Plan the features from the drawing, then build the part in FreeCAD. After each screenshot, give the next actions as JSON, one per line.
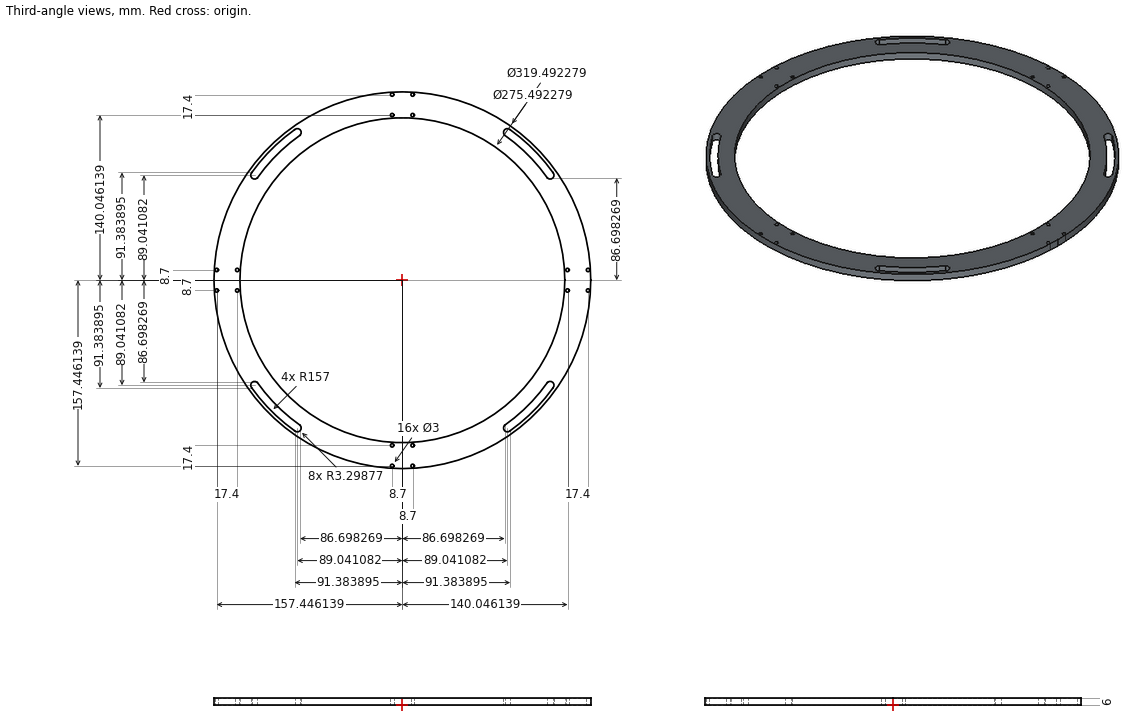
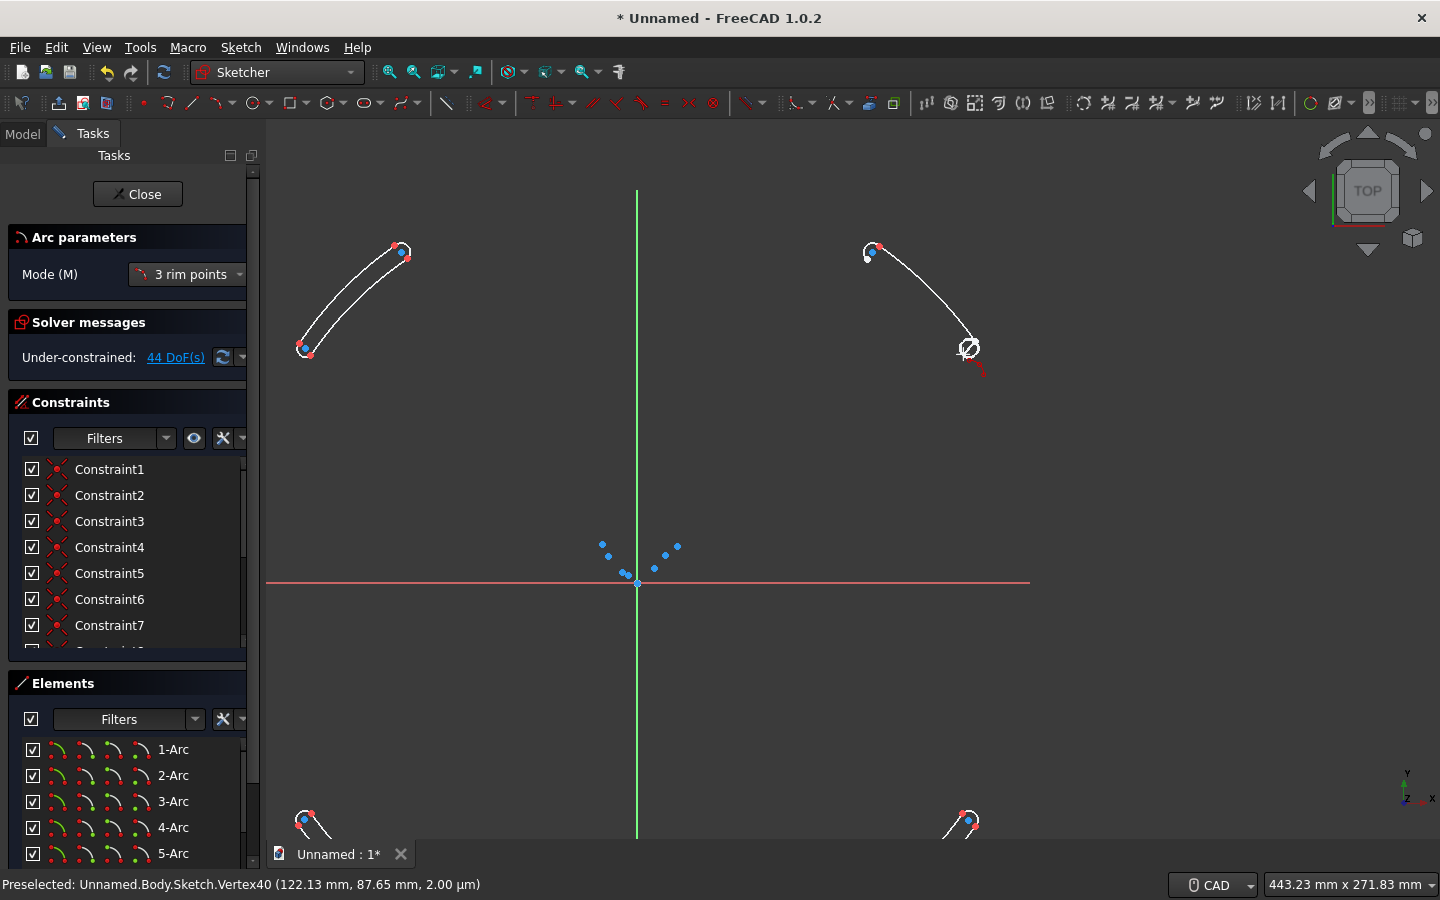
{"action": "scroll", "coordinate": [975, 354], "scroll_direction": "up", "scroll_amount": 3}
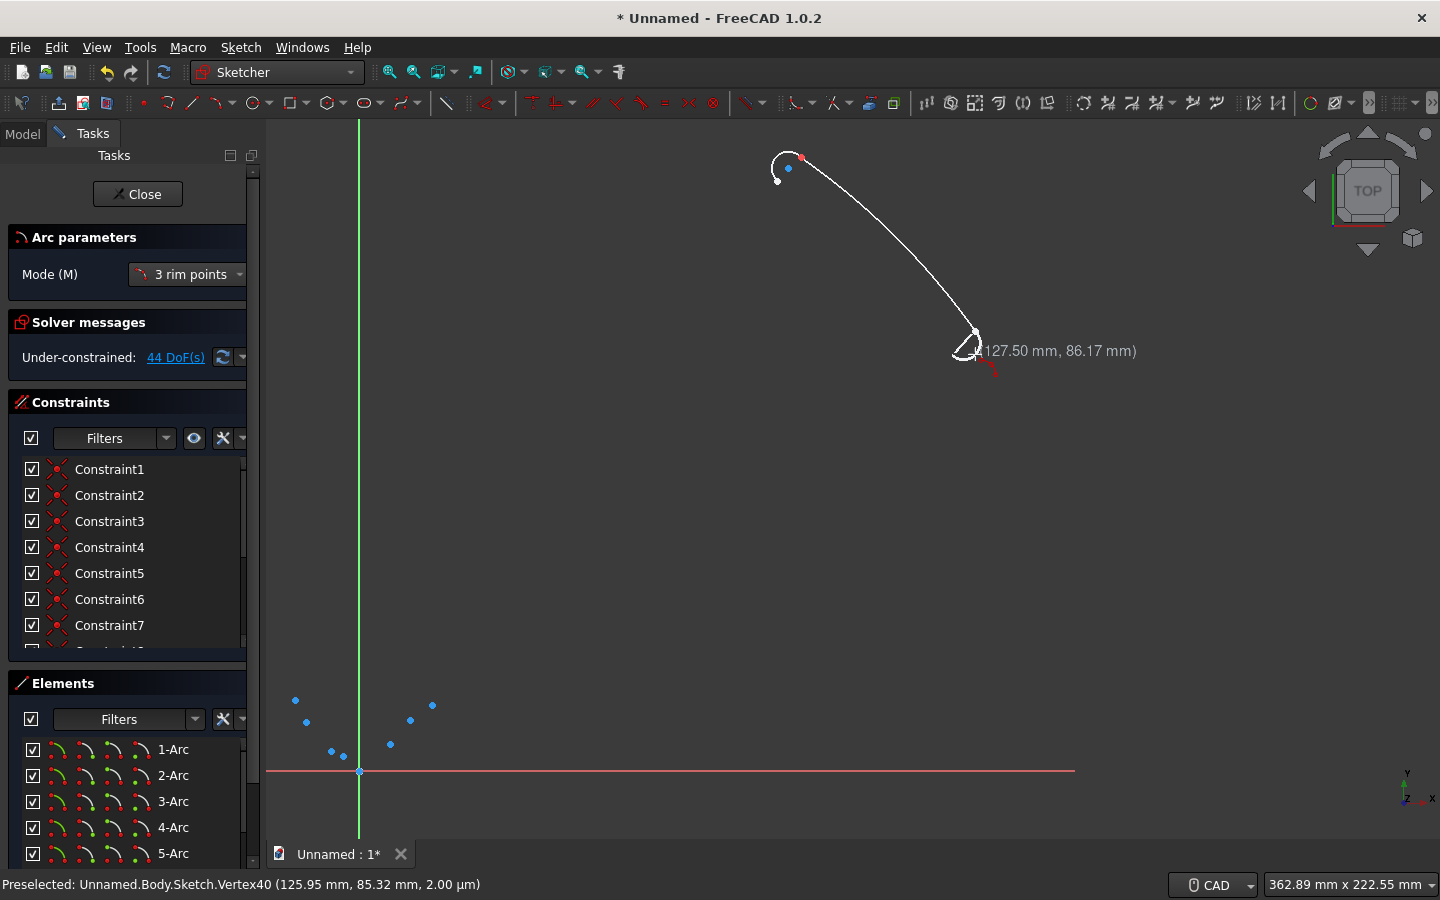
{"action": "left_click", "coordinate": [975, 353]}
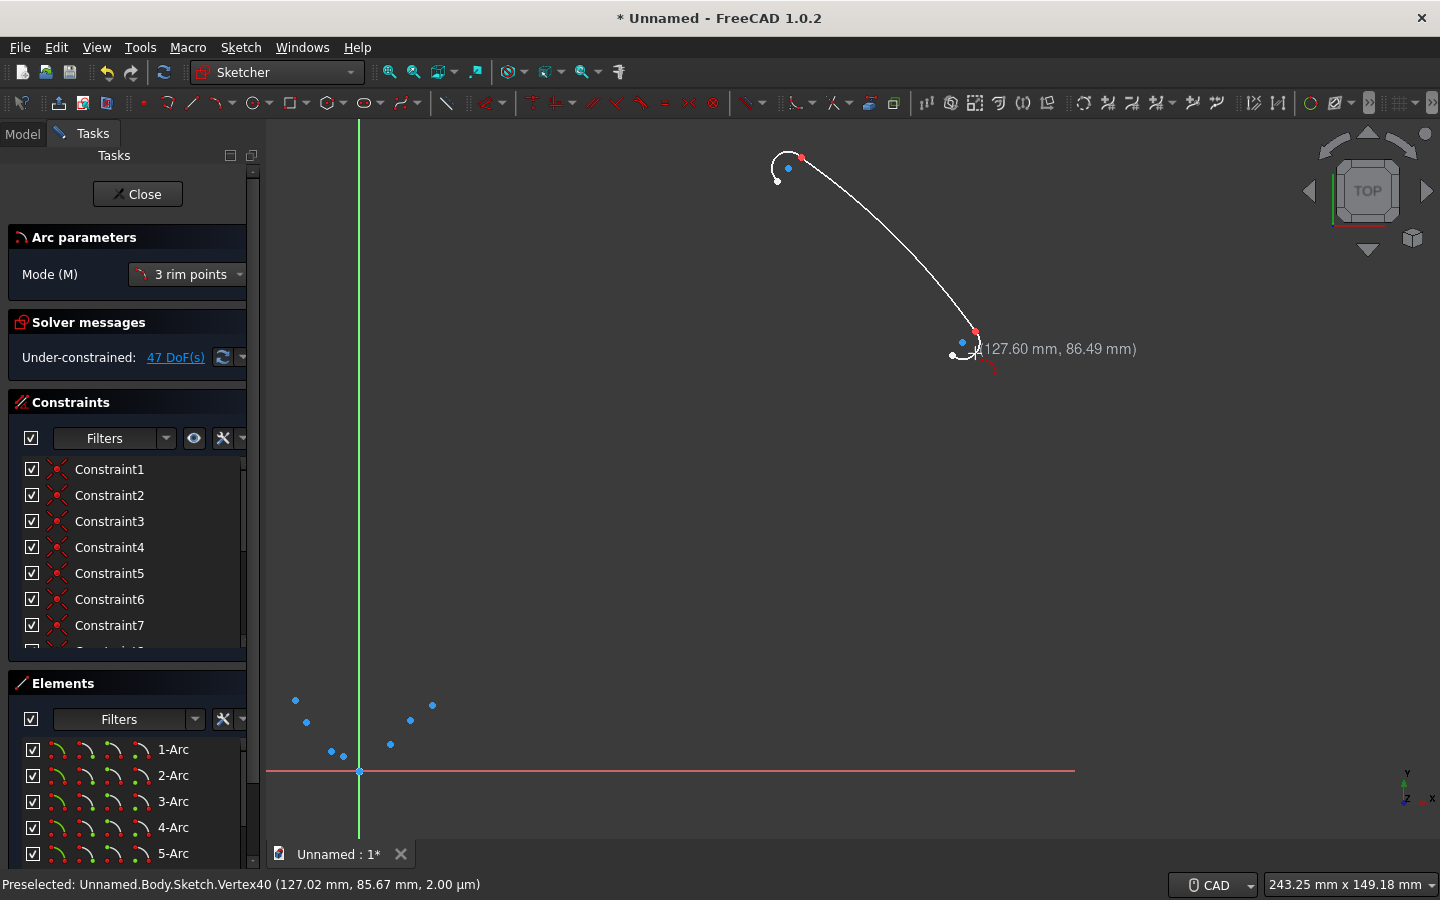
{"action": "left_click", "coordinate": [953, 356]}
{"action": "left_click", "coordinate": [778, 181]}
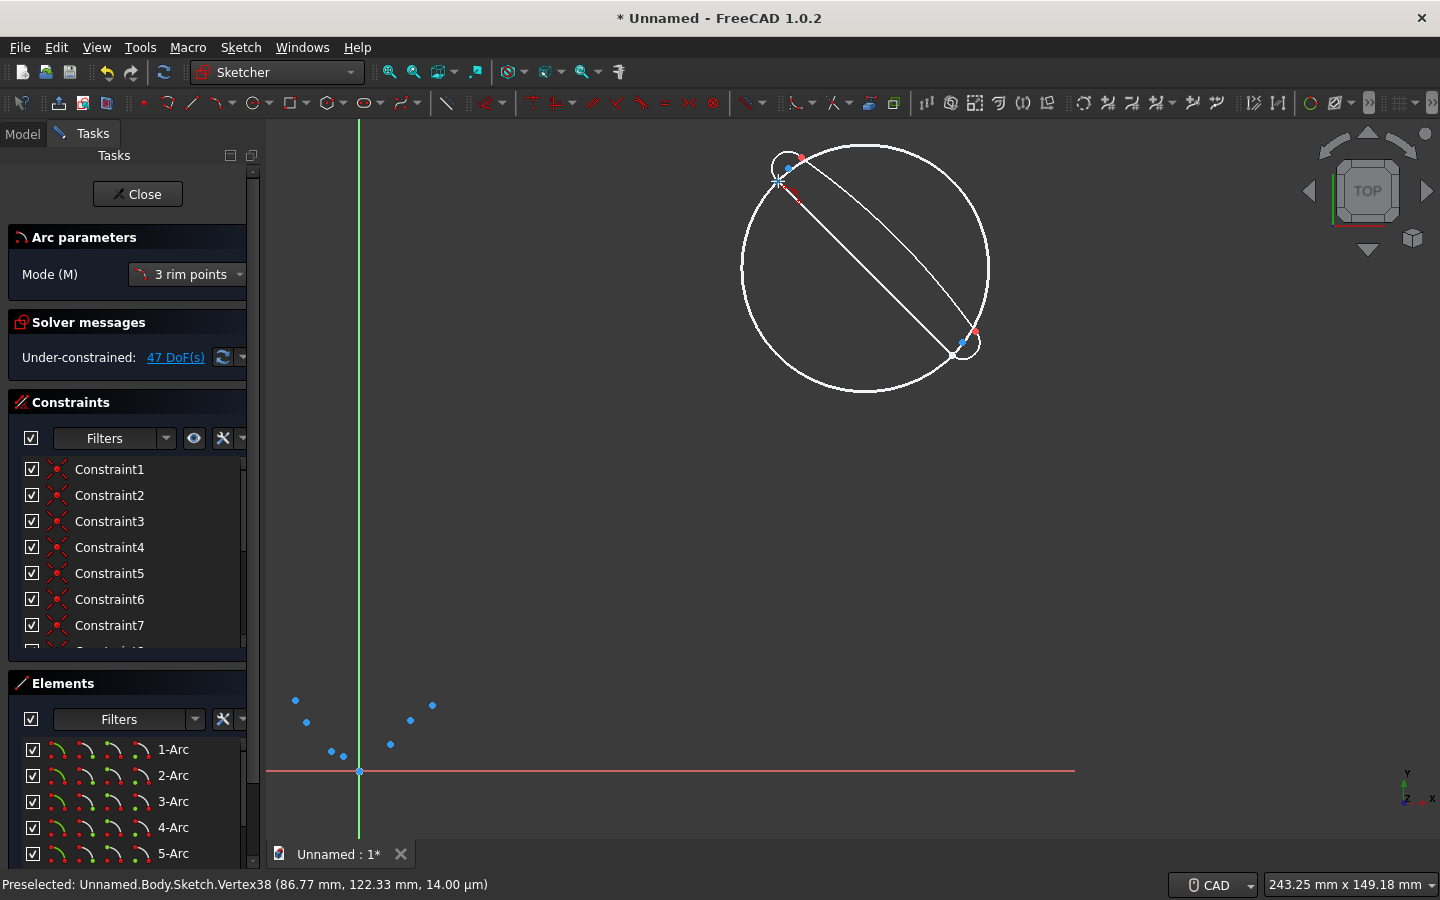
{"action": "scroll", "coordinate": [873, 258], "scroll_direction": "up", "scroll_amount": 2}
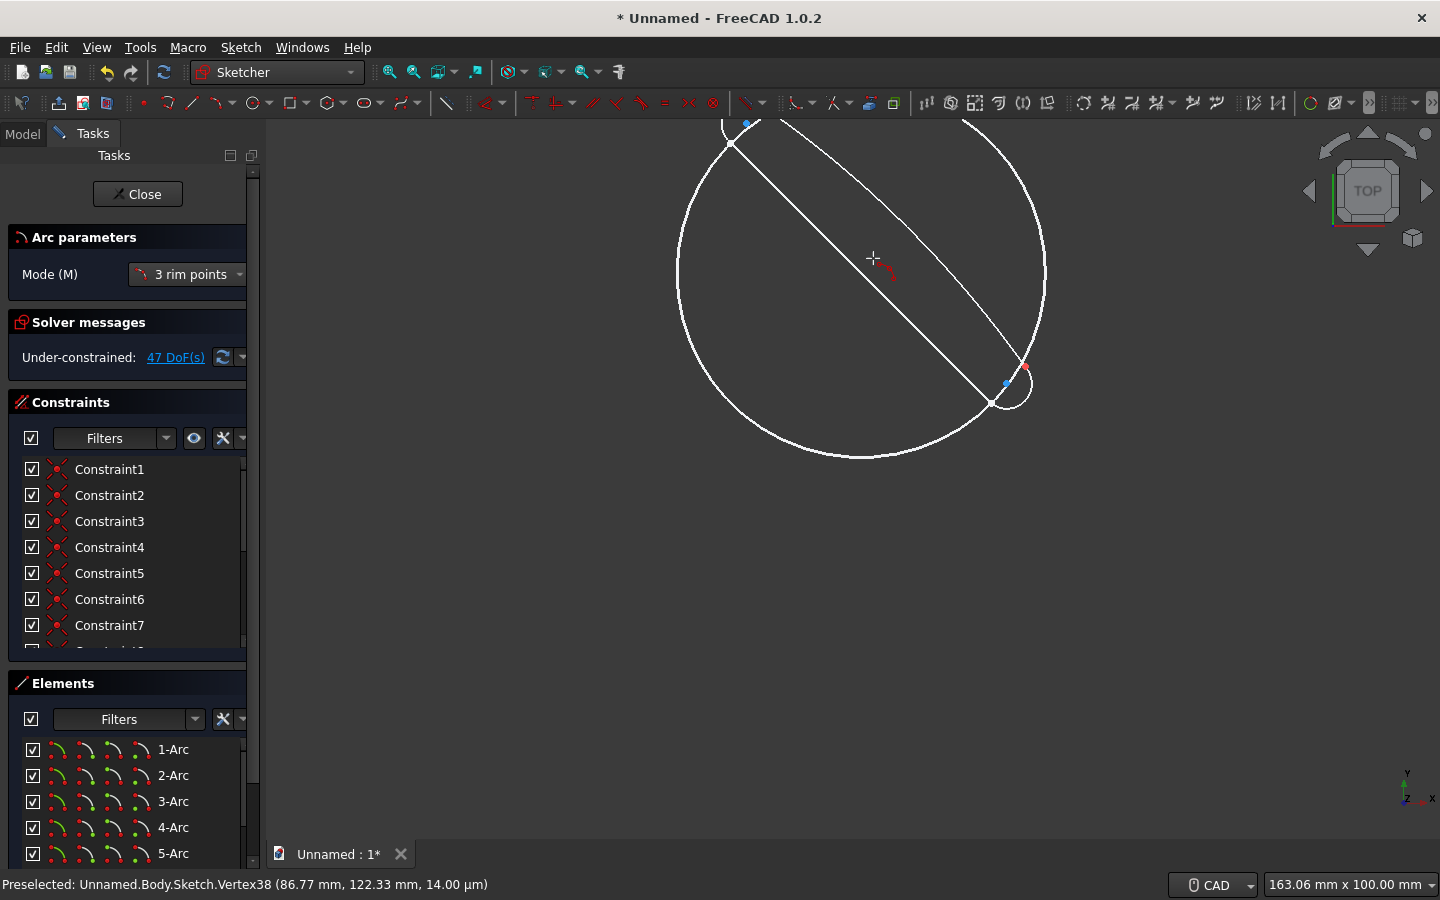
{"action": "left_click", "coordinate": [872, 258]}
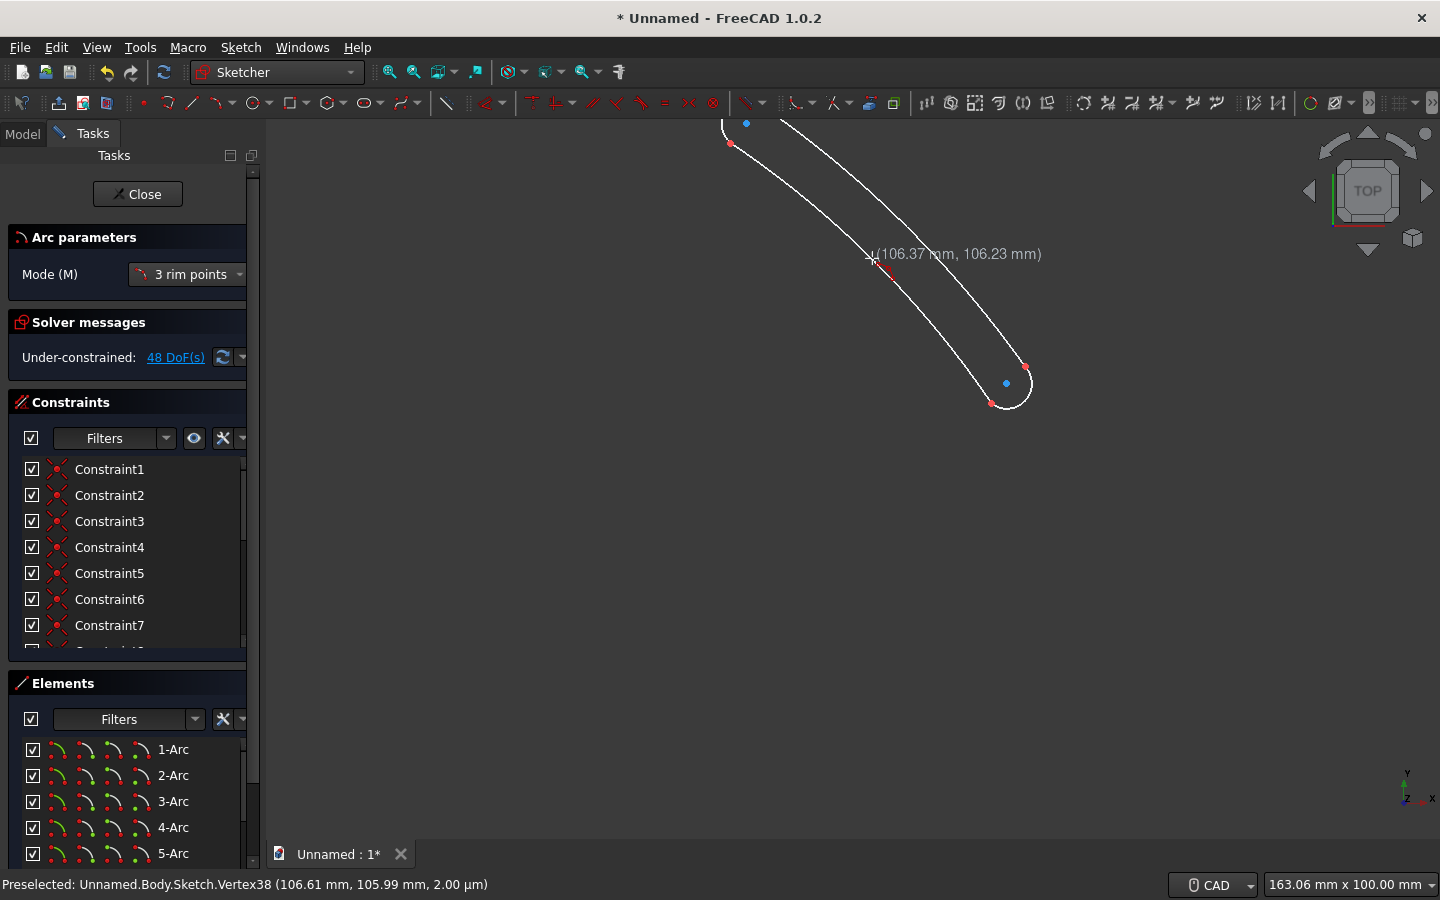
{"action": "key", "text": "g c"}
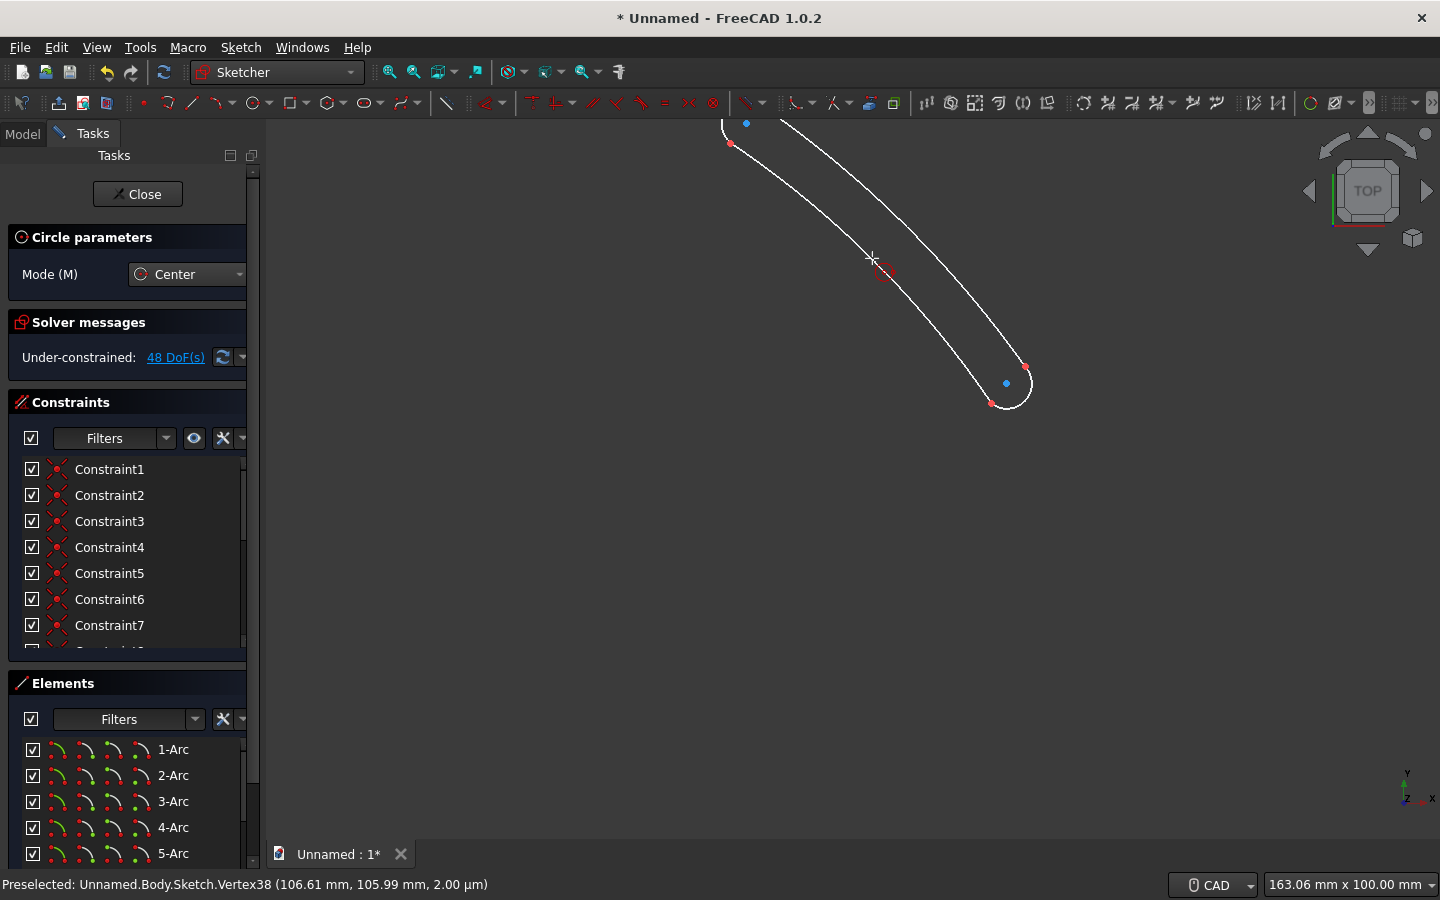
{"action": "scroll", "coordinate": [956, 341], "scroll_direction": "down", "scroll_amount": 8}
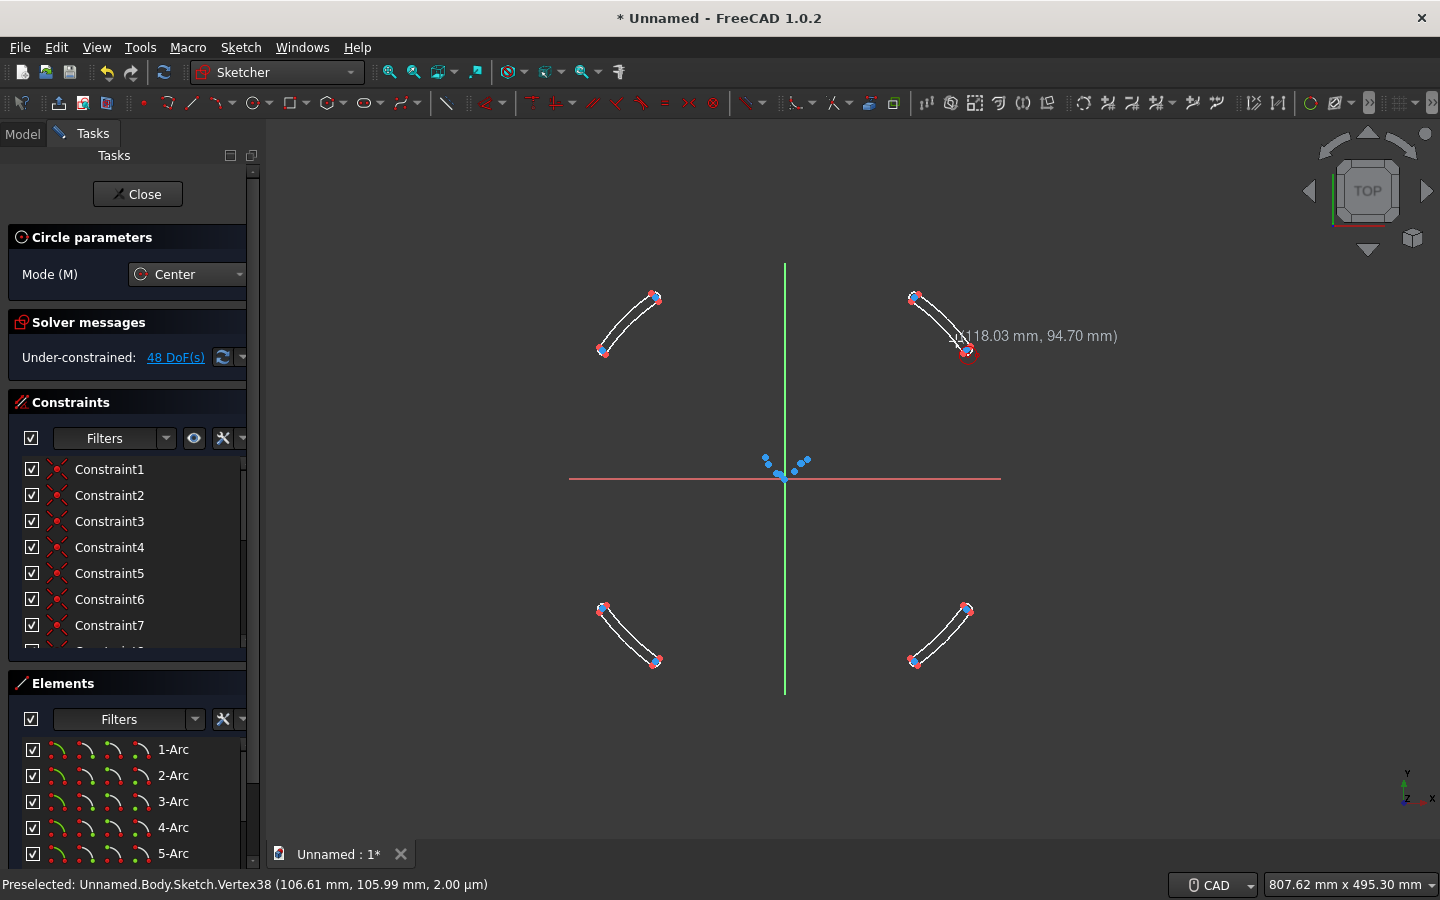
{"action": "left_click", "coordinate": [785, 479]}
{"action": "mouse_move", "coordinate": [1003, 400]}